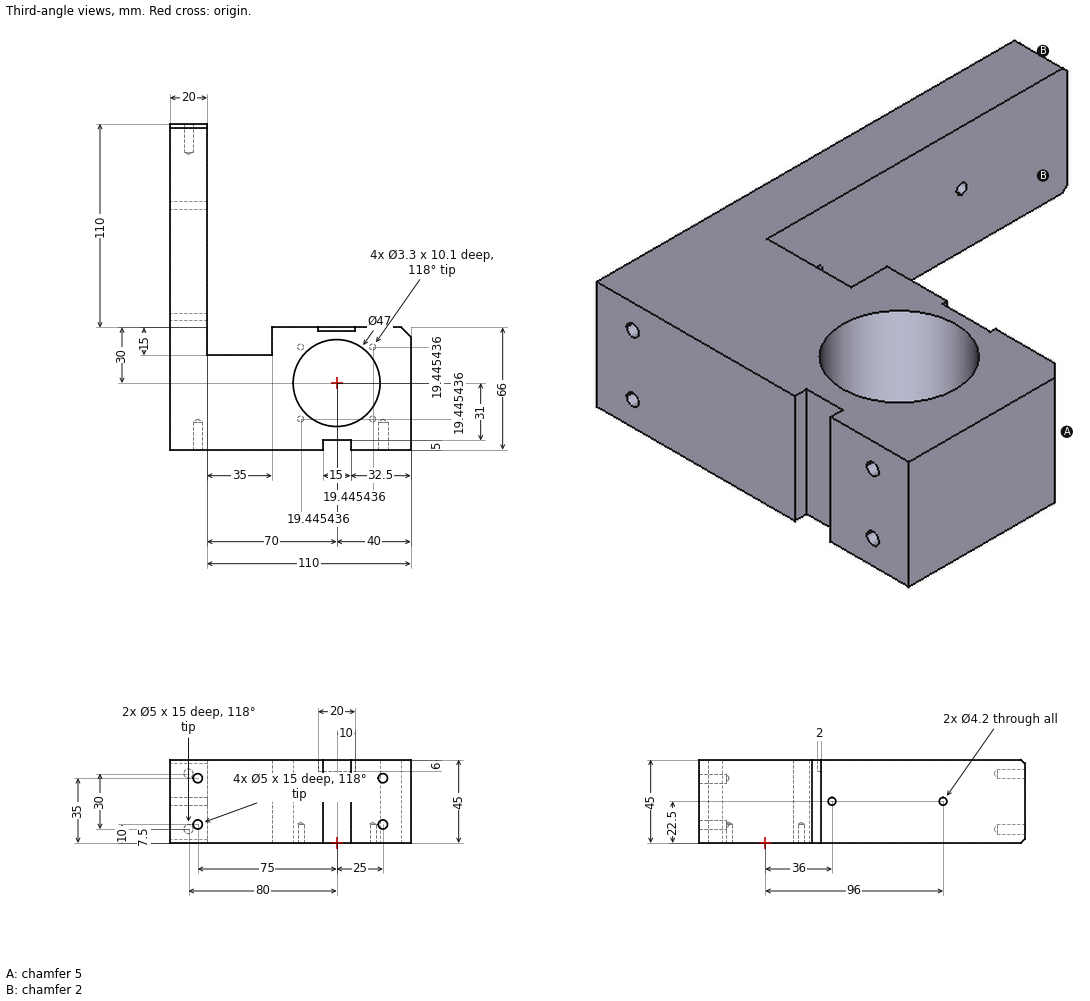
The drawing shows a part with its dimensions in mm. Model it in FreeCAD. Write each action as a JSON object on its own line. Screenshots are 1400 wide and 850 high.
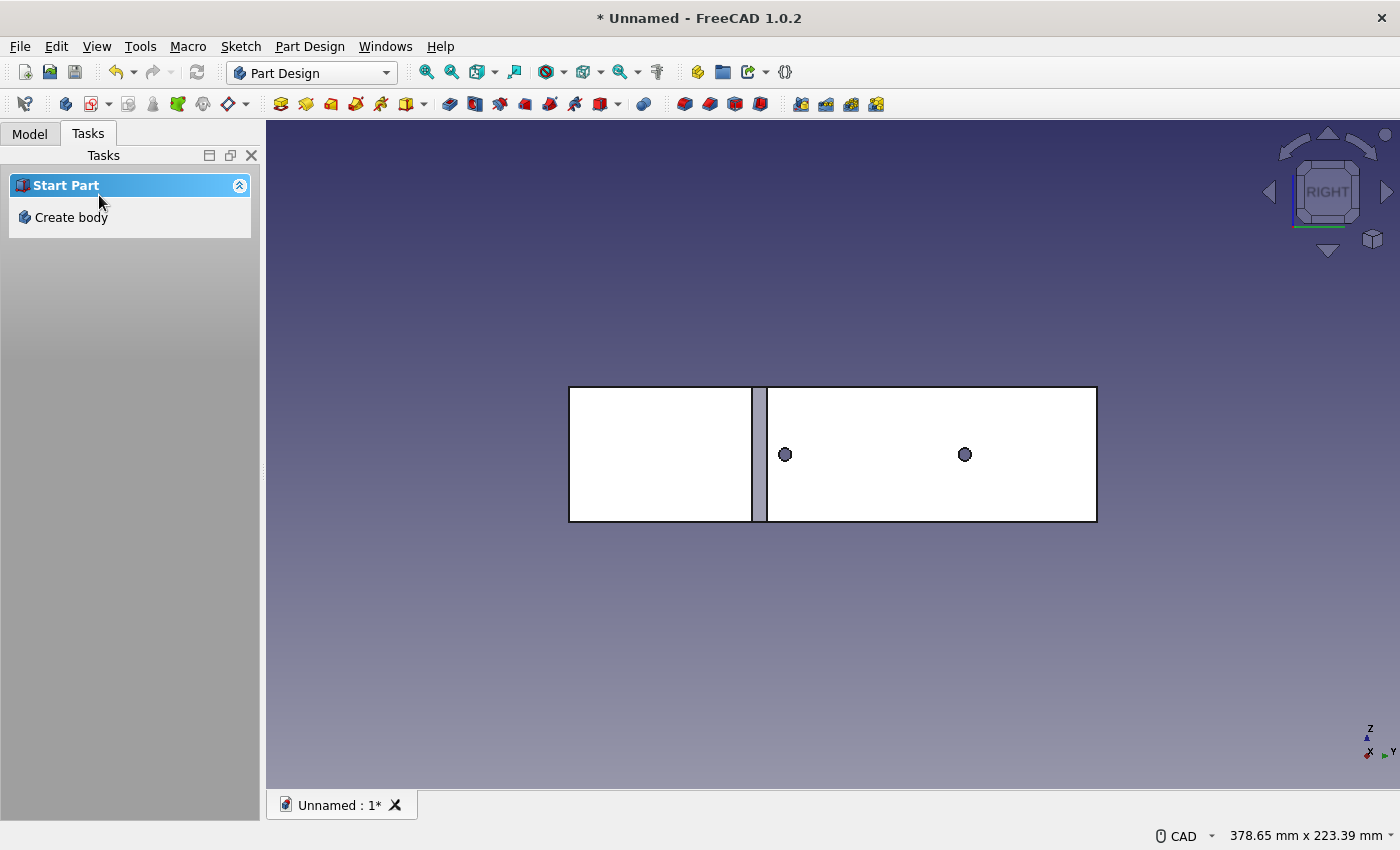
{"action": "key", "text": "0"}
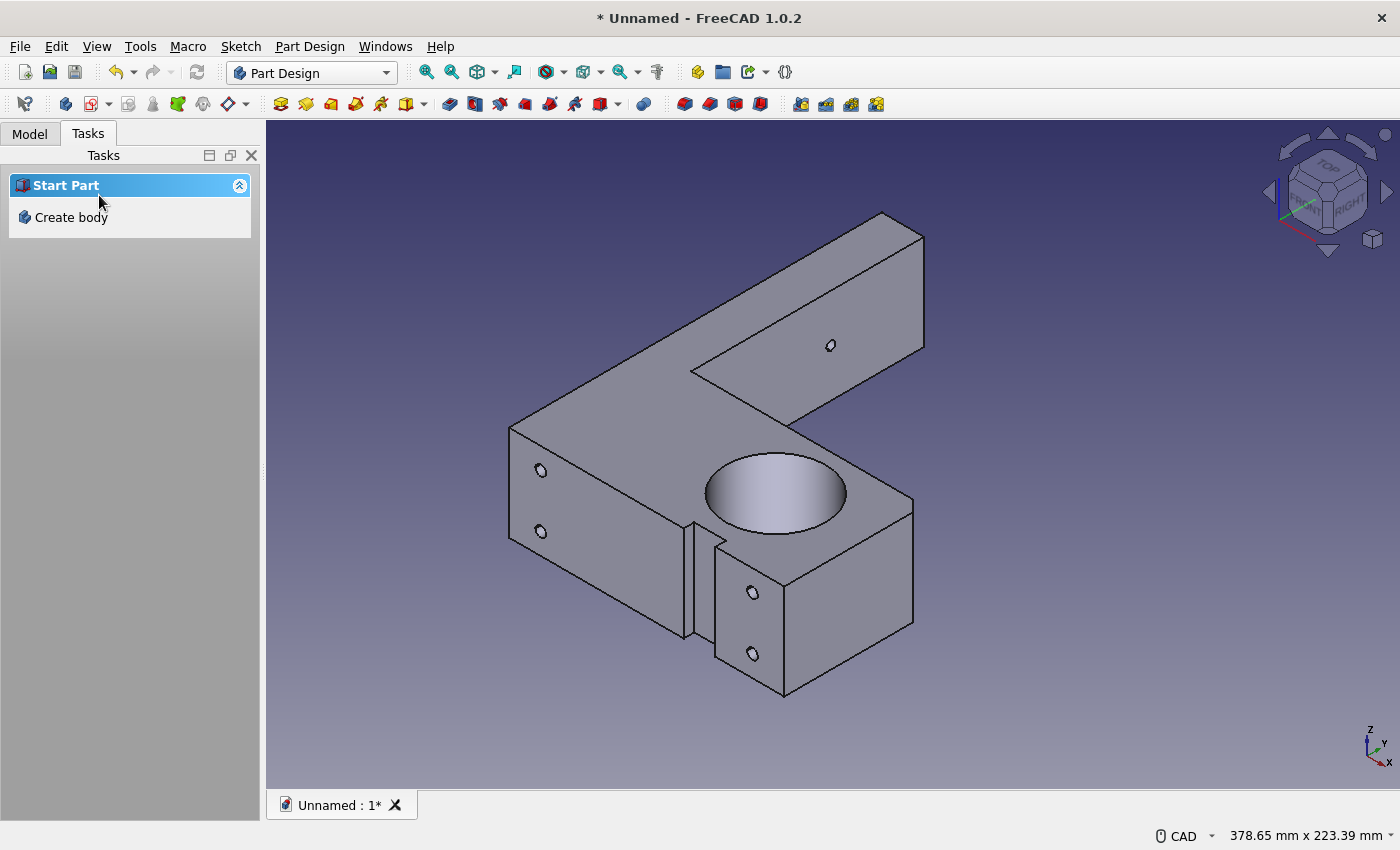
{"action": "key", "text": "2"}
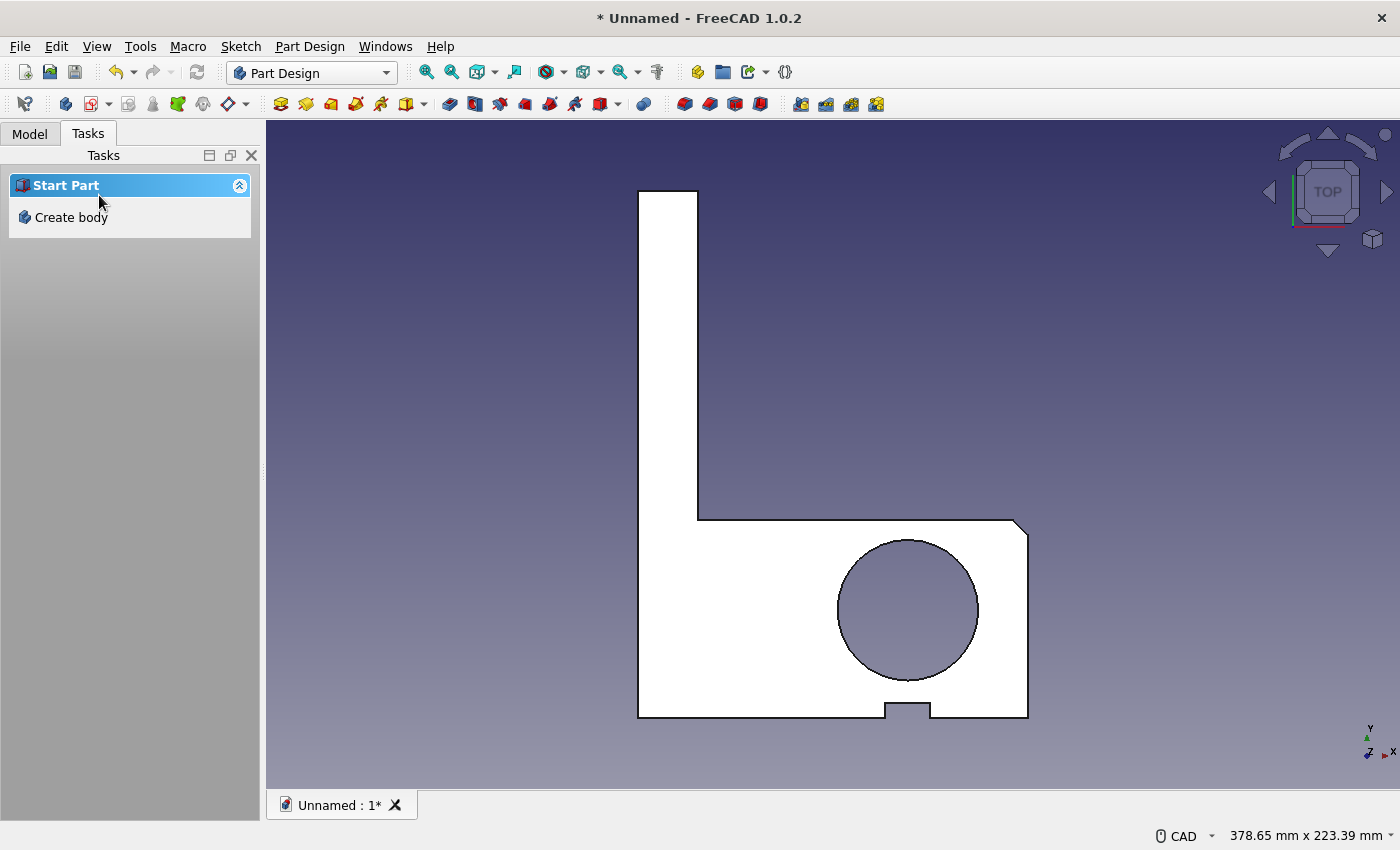
{"action": "left_click", "coordinate": [668, 190]}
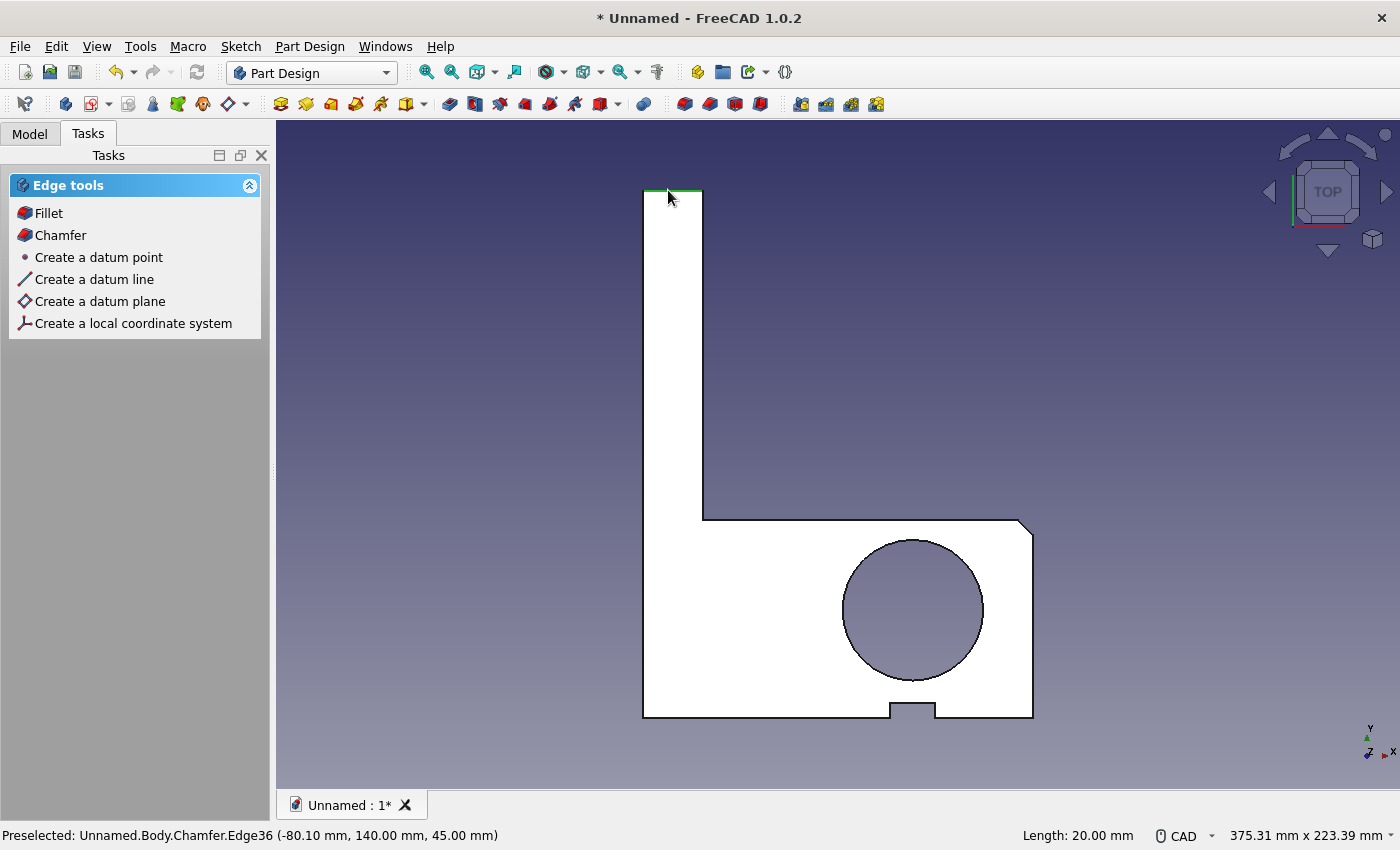
{"action": "key", "text": "1"}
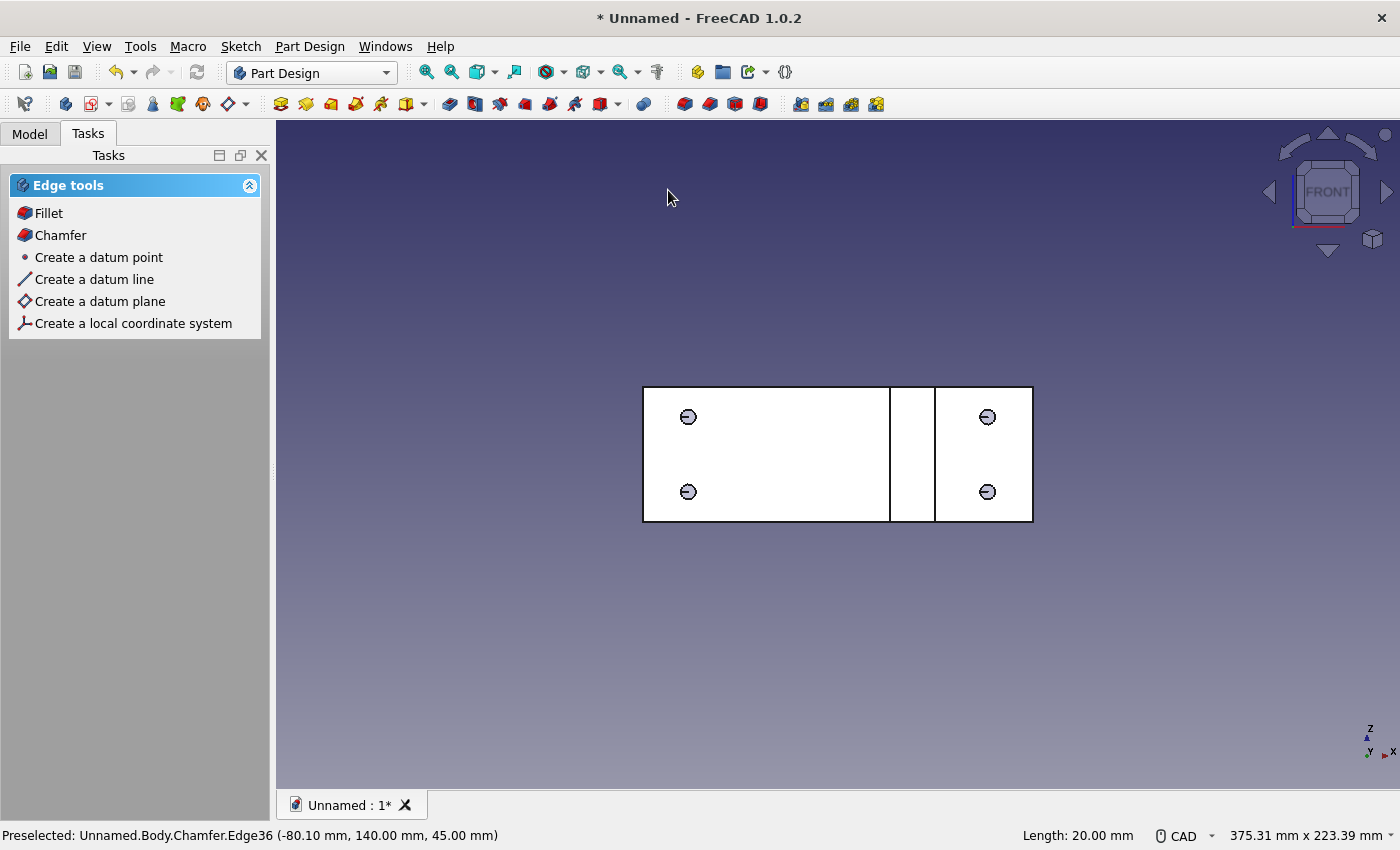
{"action": "left_click", "coordinate": [427, 72]}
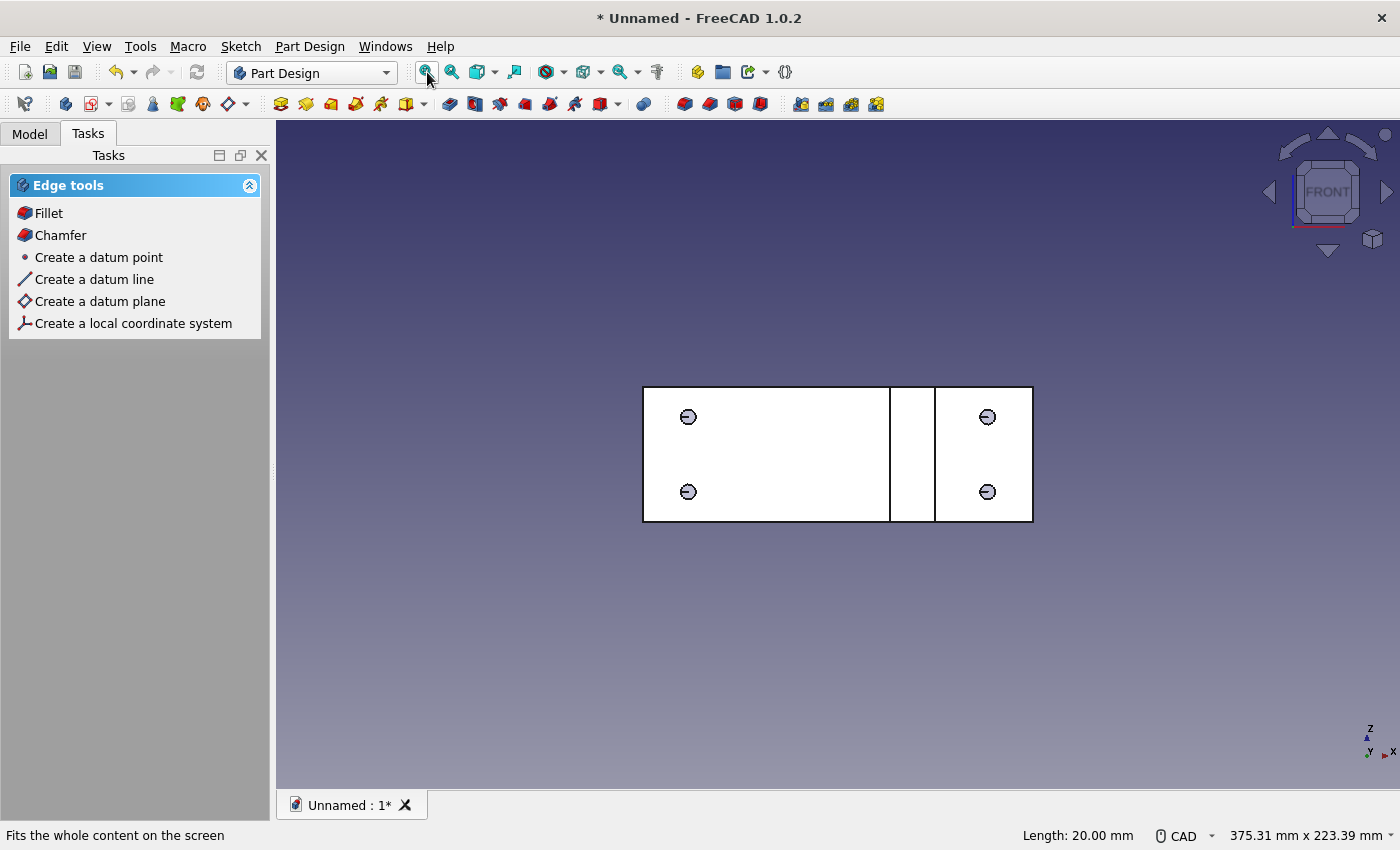
{"action": "key", "text": "3"}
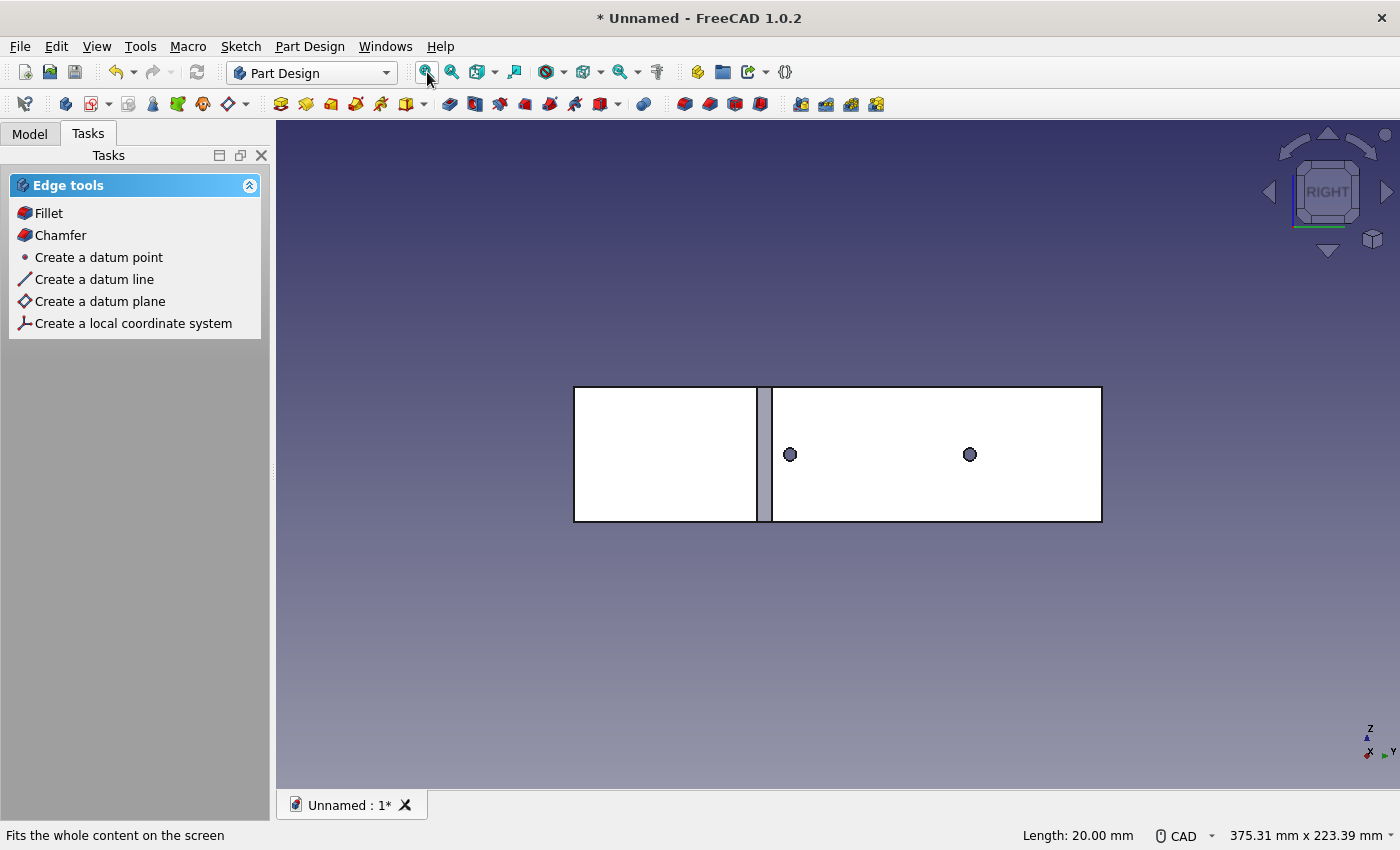
{"action": "key", "text": "5"}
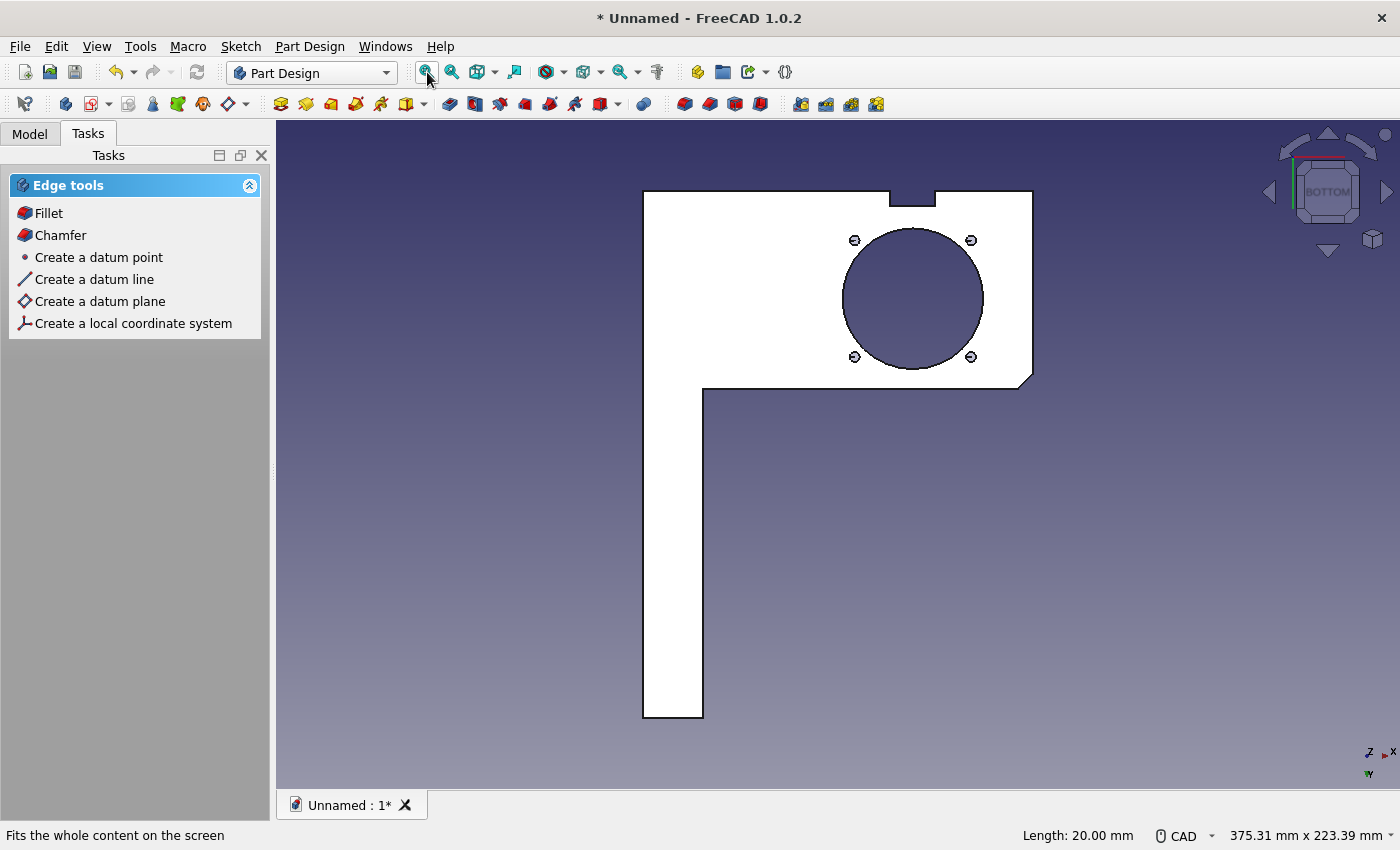
{"action": "left_click", "coordinate": [673, 717], "text": "ctrl"}